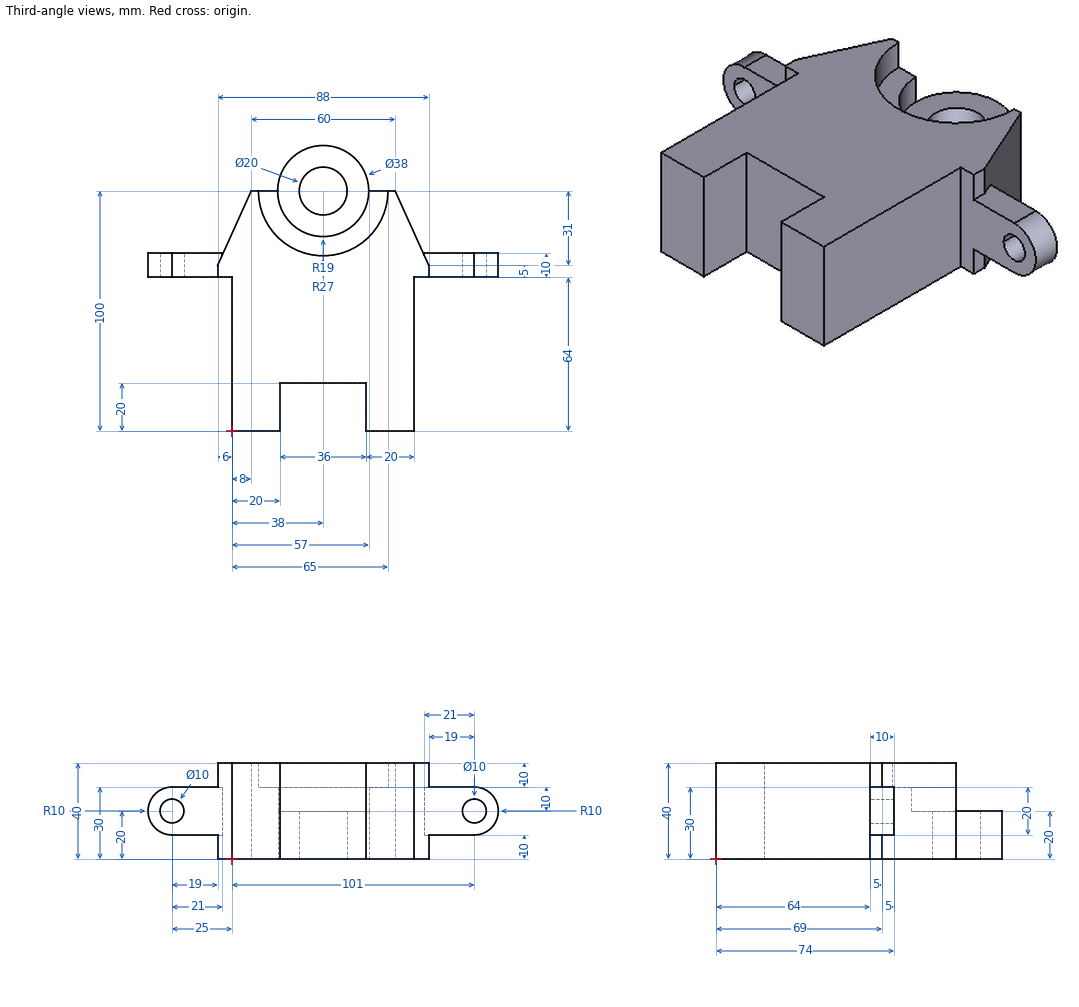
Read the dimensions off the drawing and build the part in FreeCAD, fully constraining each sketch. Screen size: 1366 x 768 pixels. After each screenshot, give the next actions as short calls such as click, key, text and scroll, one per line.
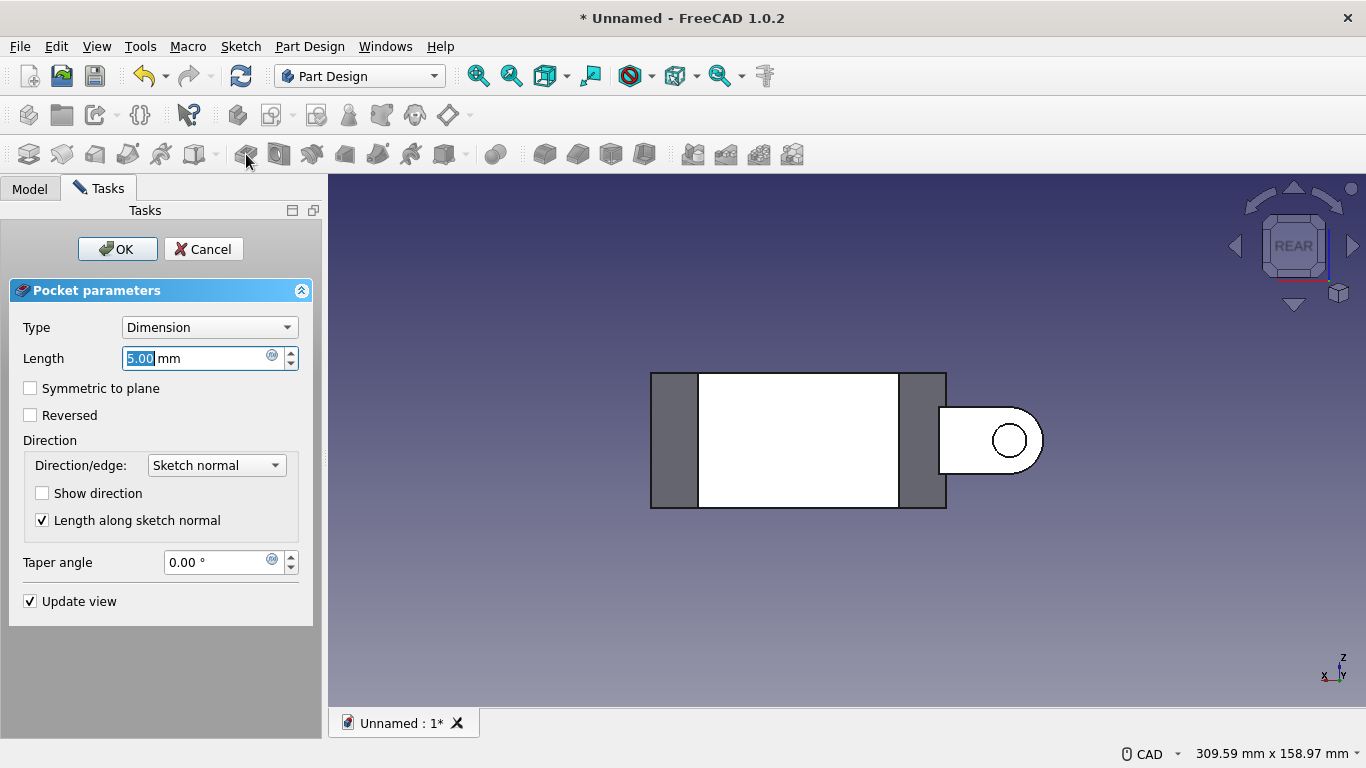
text(10)
key(Tab)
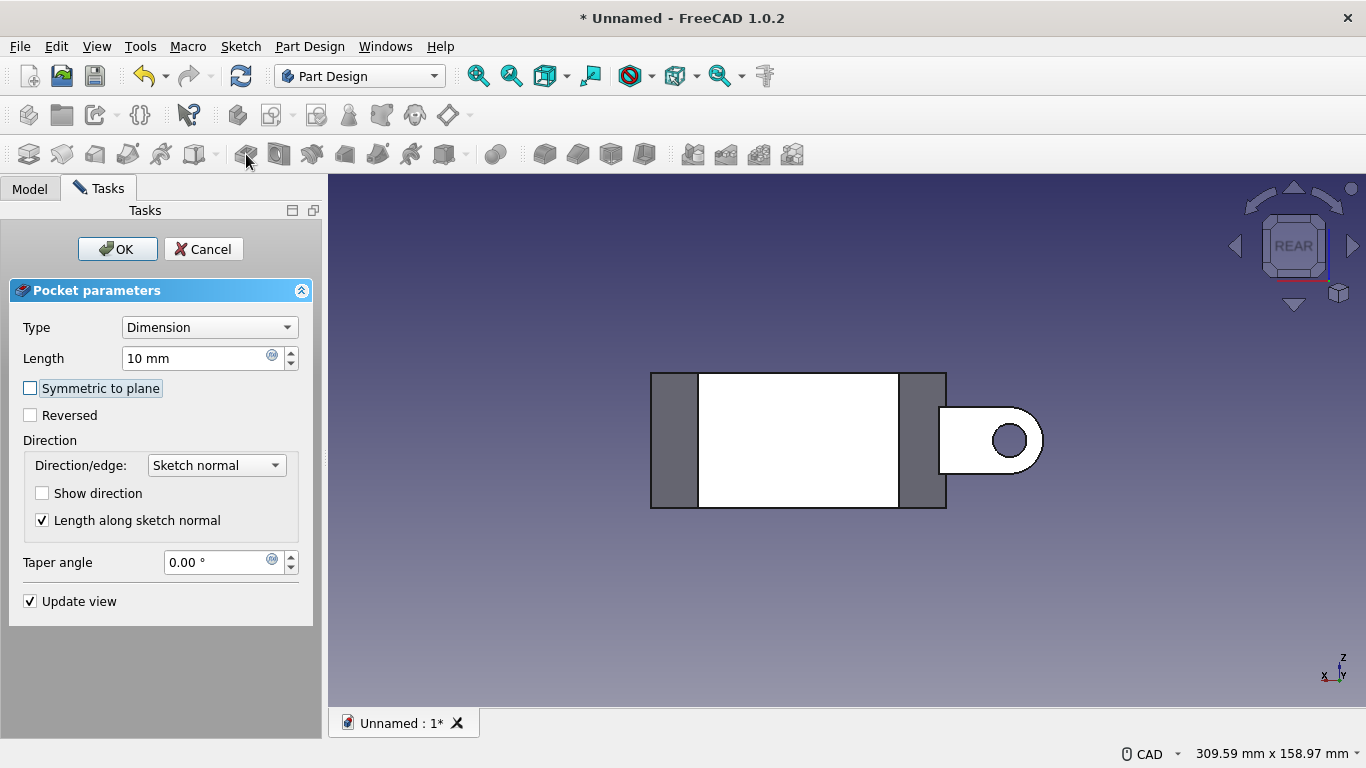
click(118, 249)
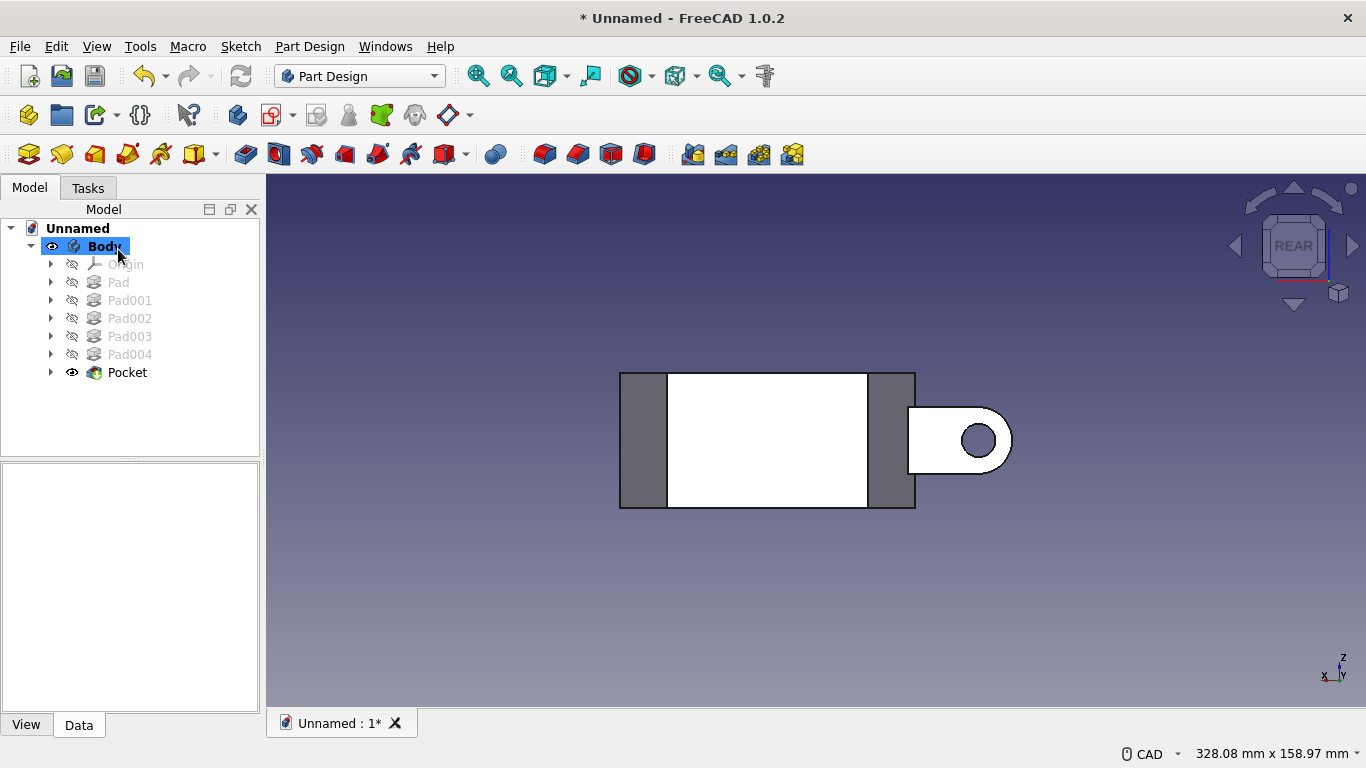
click(479, 76)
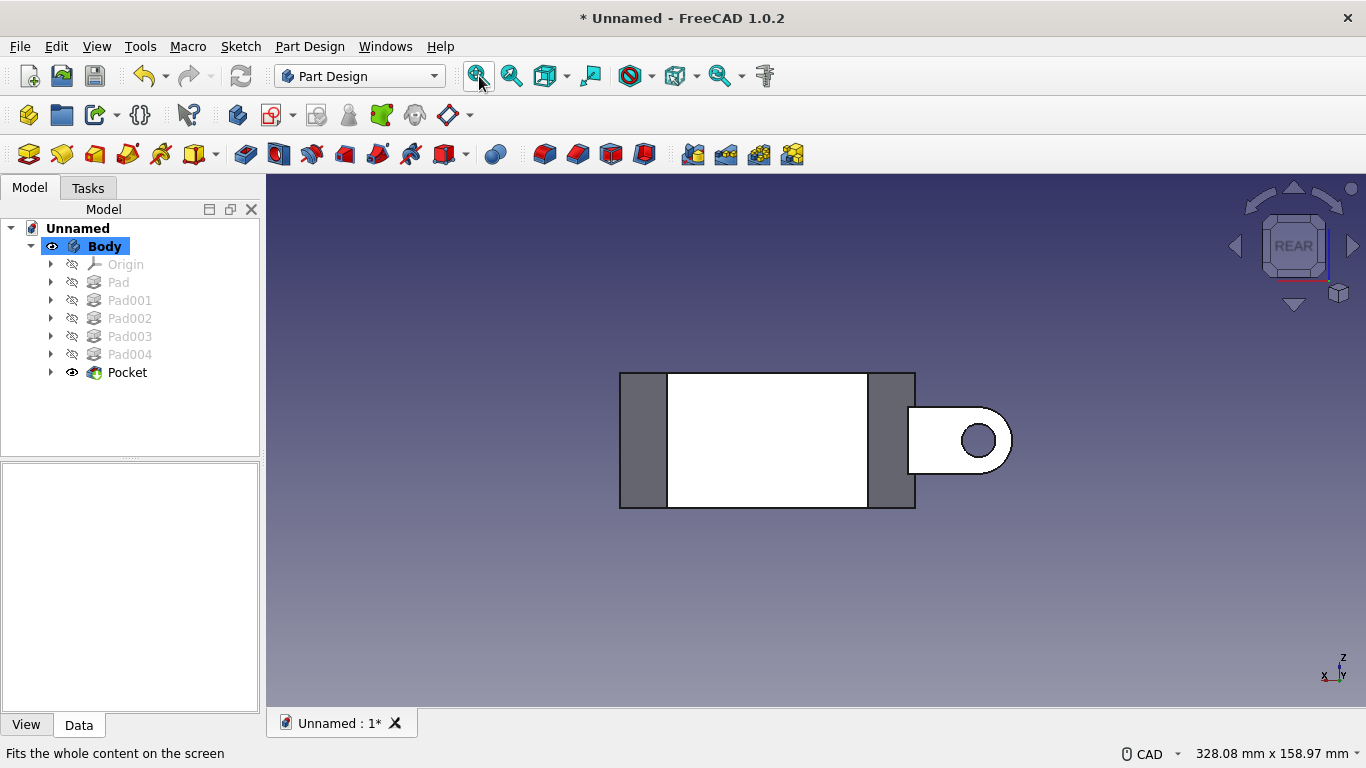
key(0)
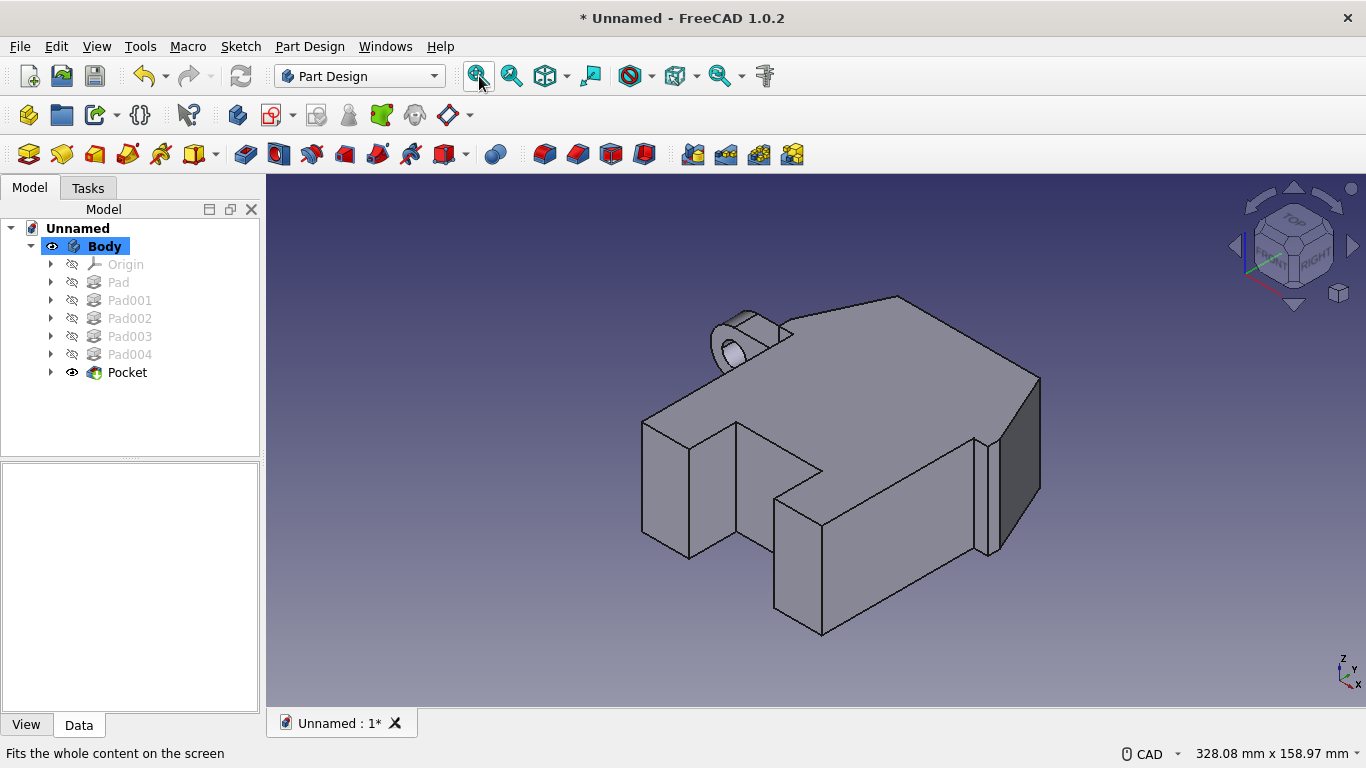
key(3)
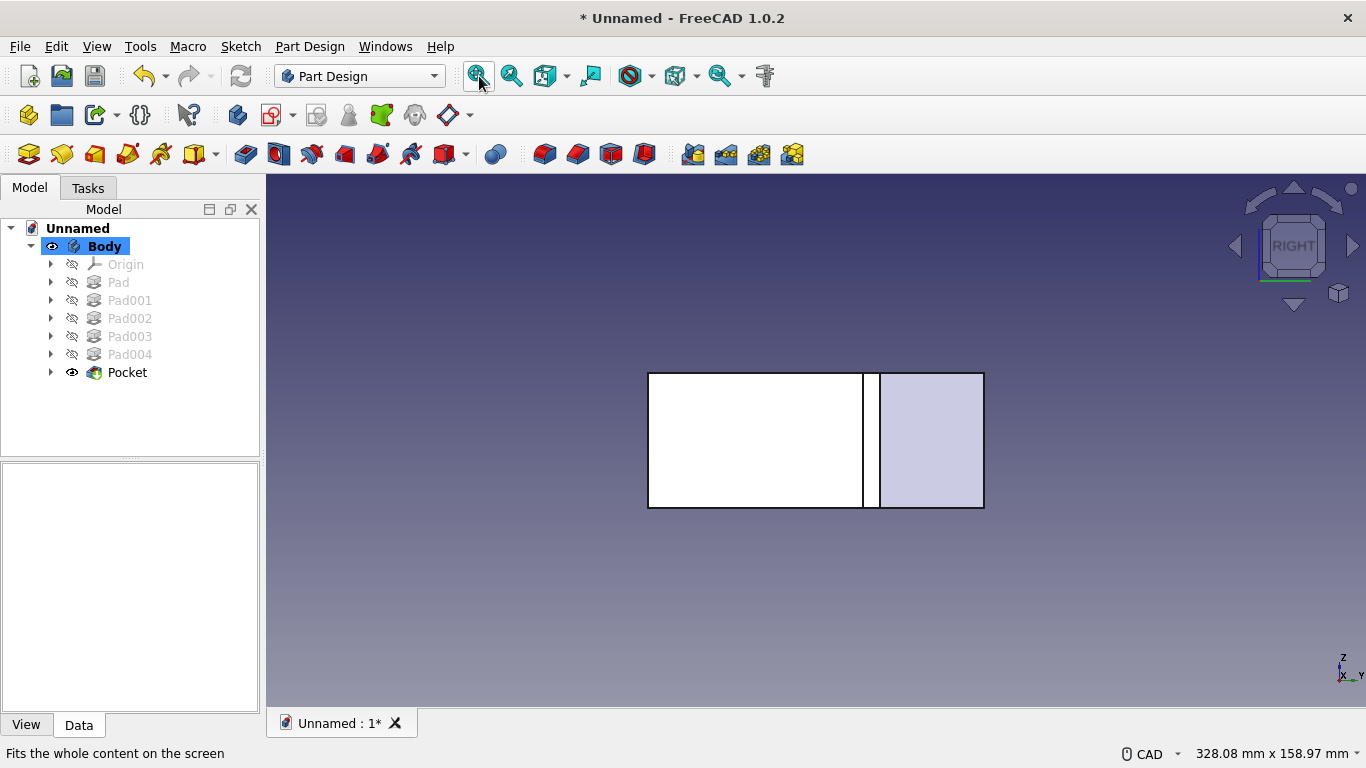
click(479, 76)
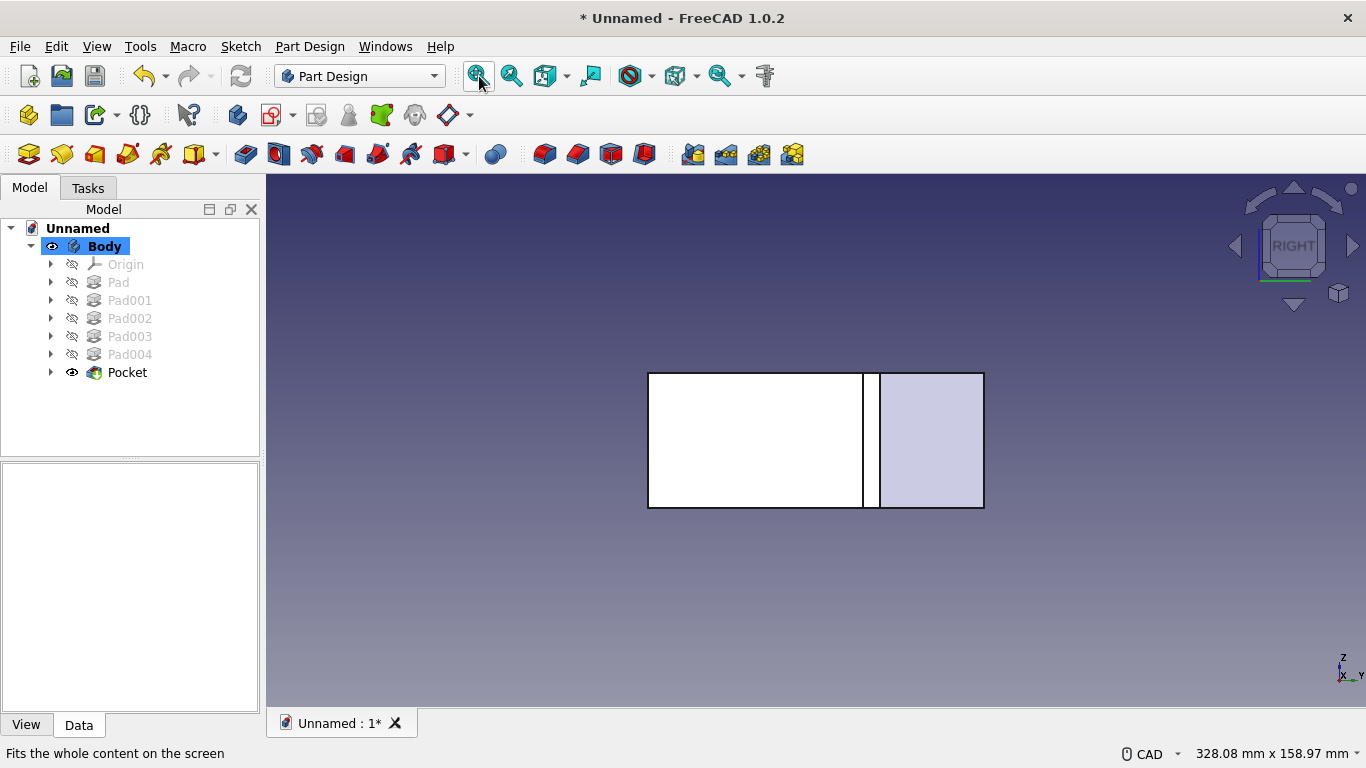
click(871, 382)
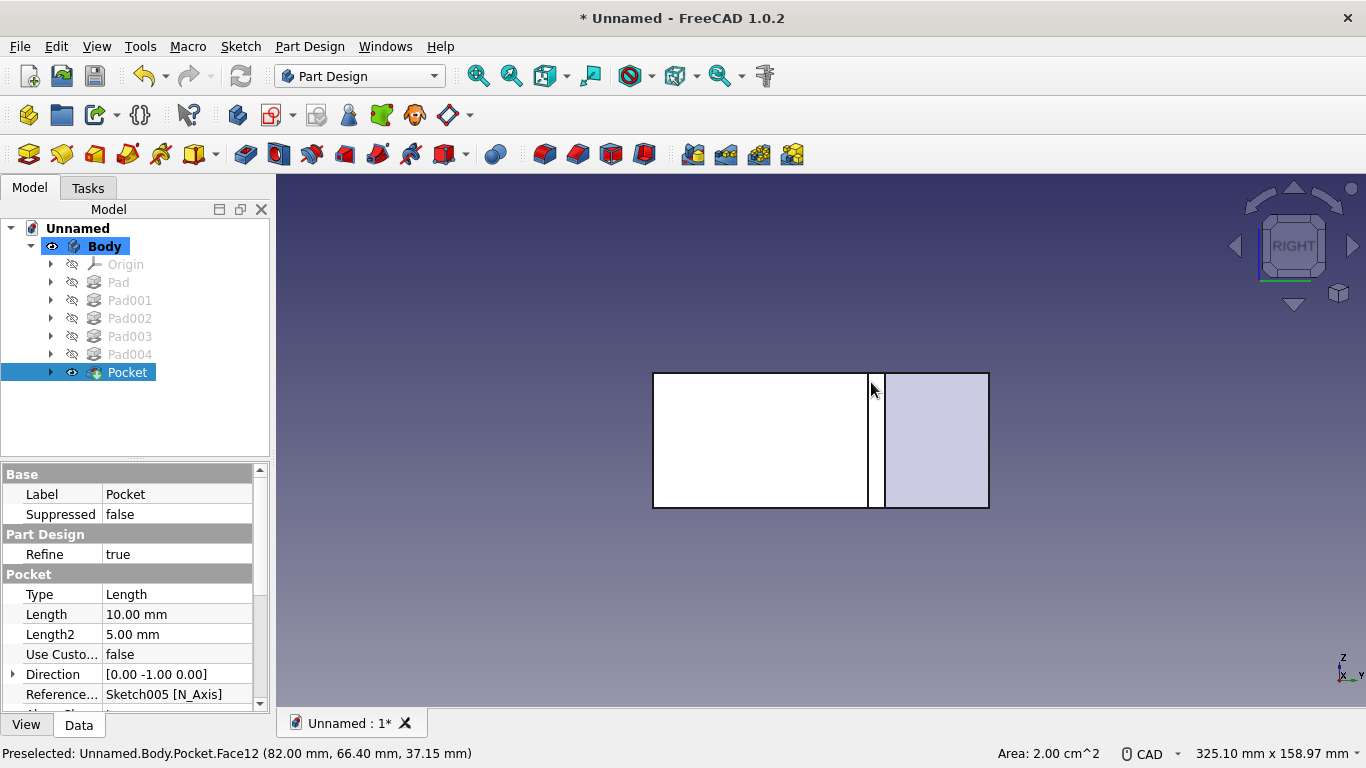
click(270, 116)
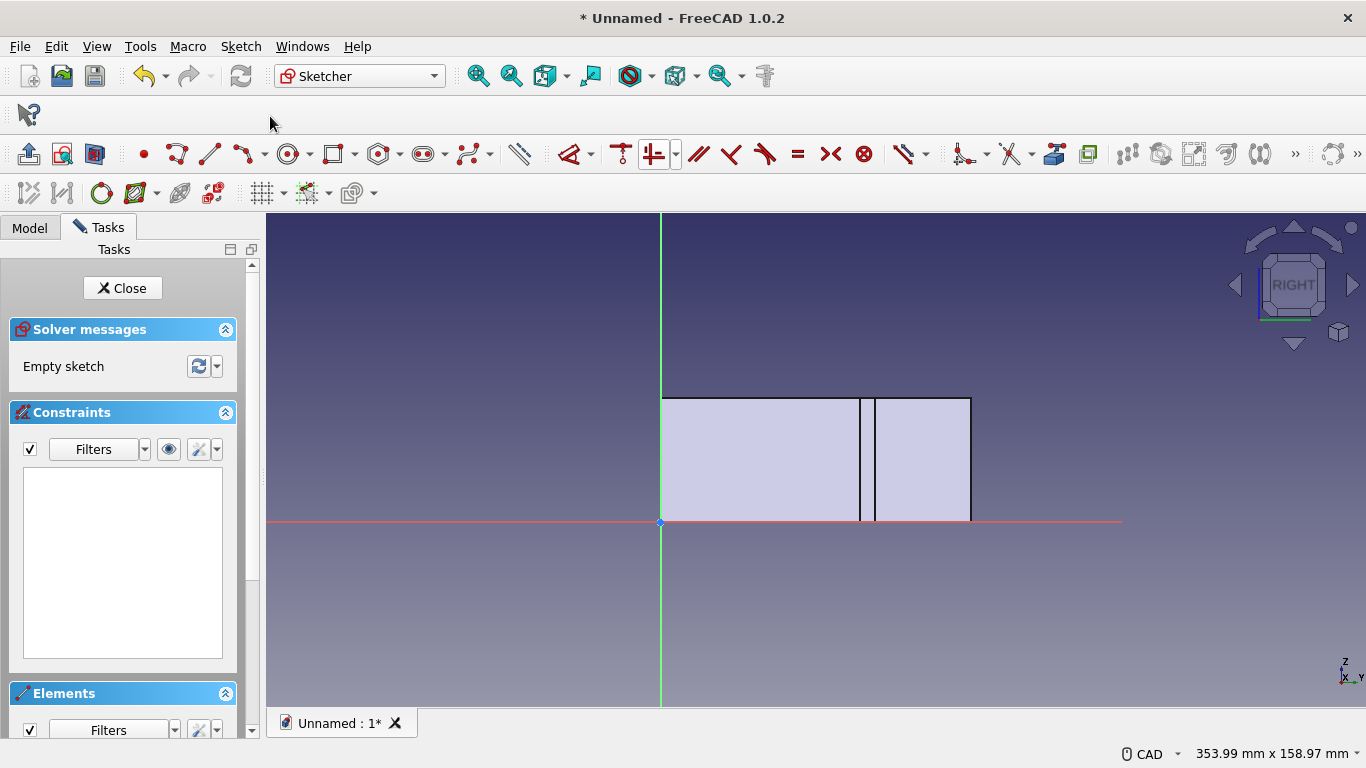
scroll(898, 460, up, 8)